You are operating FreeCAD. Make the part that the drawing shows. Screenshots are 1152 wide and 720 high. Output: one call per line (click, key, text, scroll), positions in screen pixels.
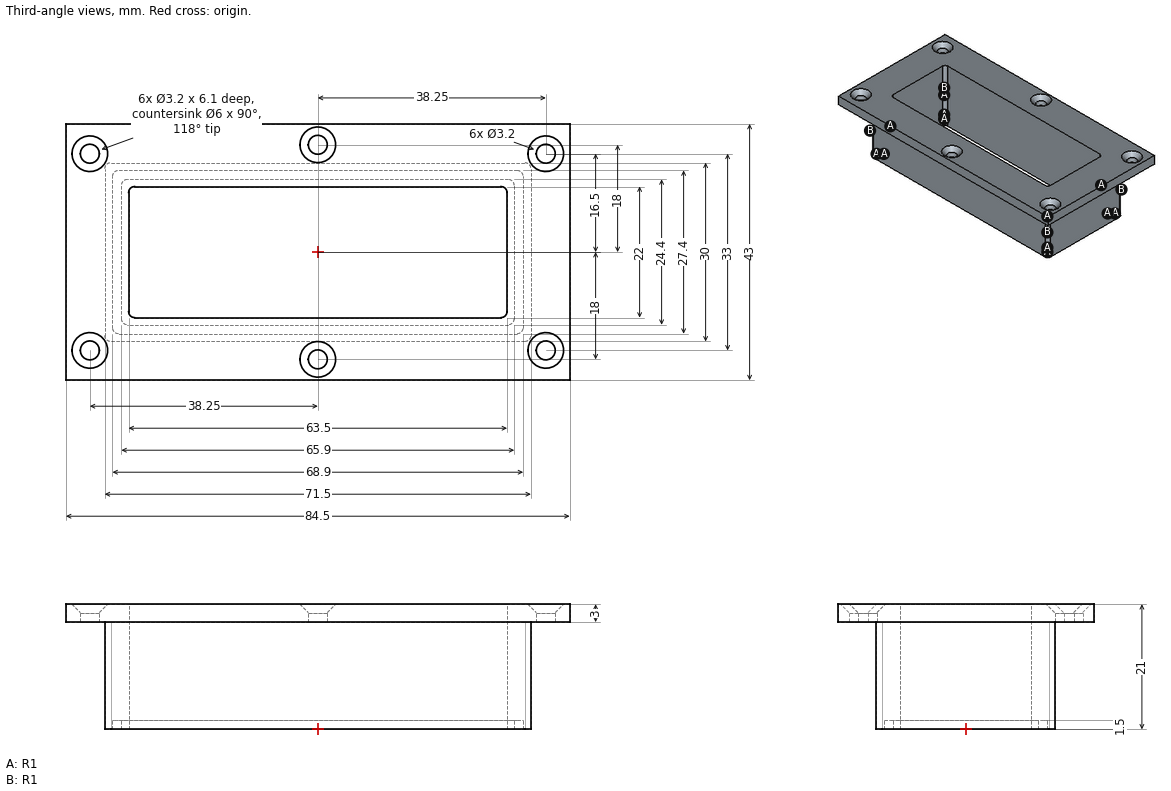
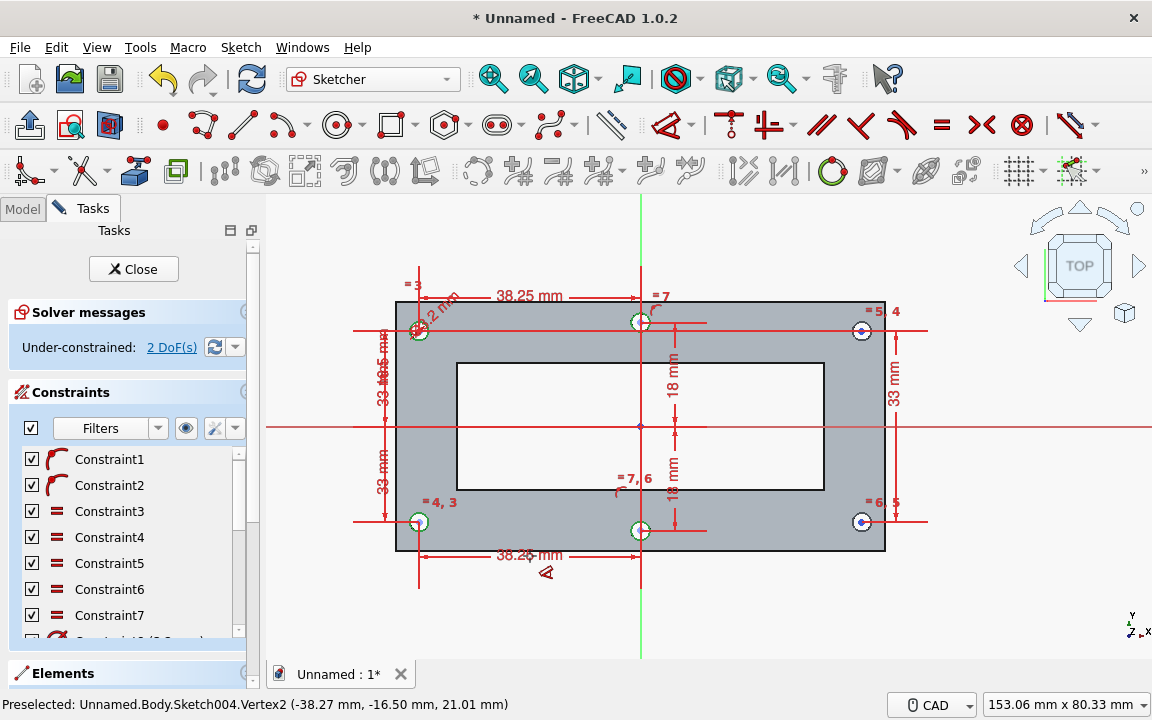
click(862, 331)
click(751, 297)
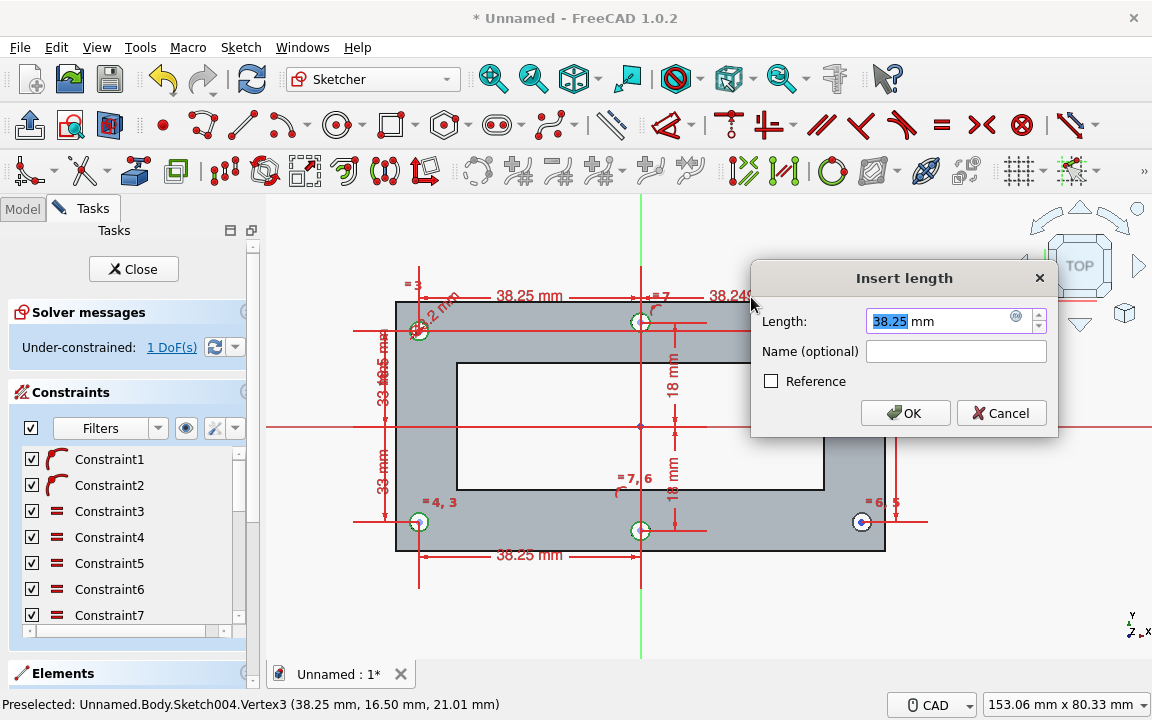
text(38.25)
key(Return)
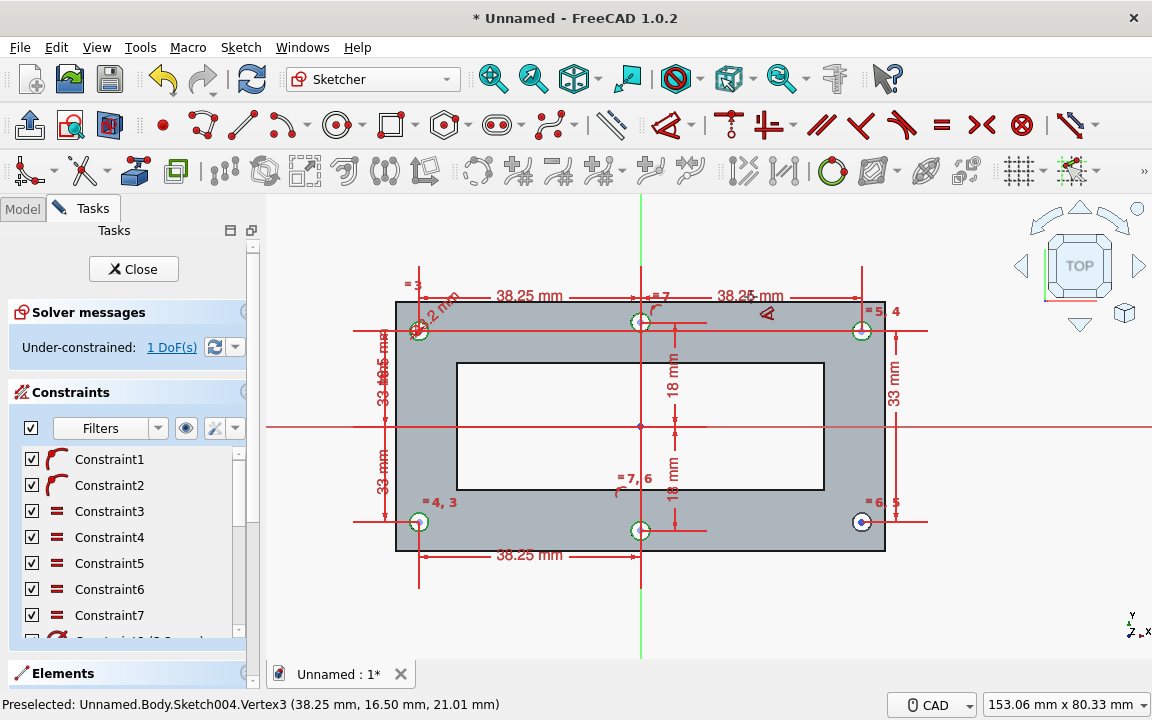
click(862, 522)
click(751, 556)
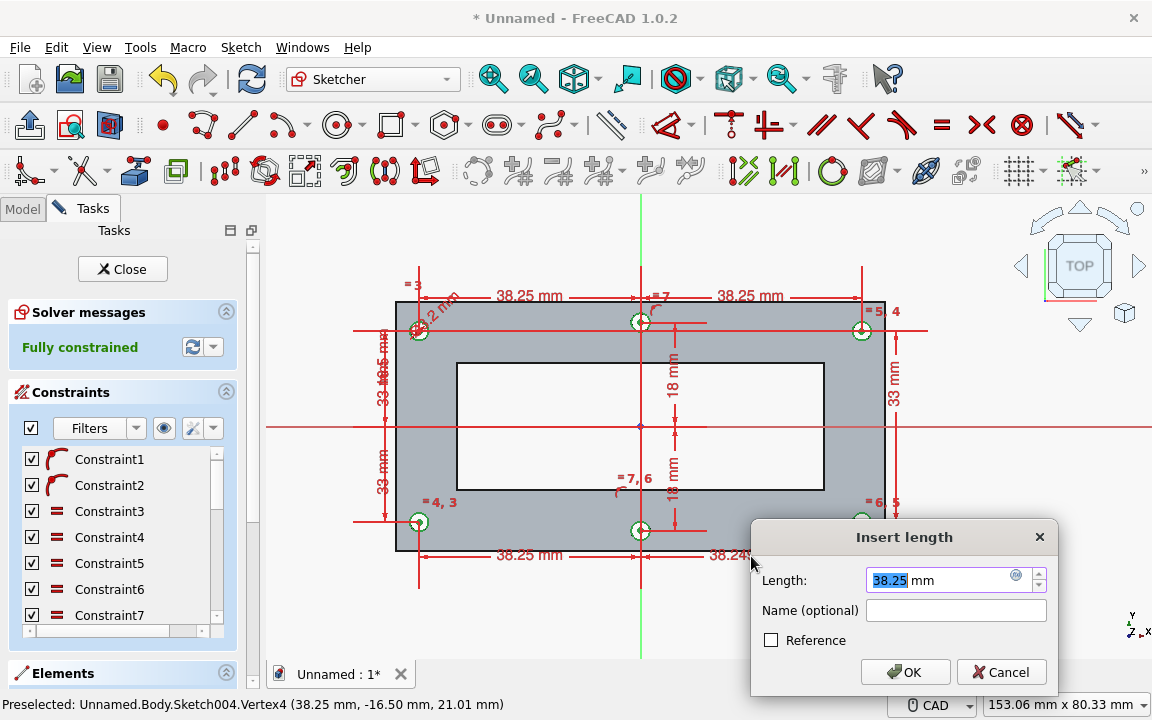
text(38.25)
key(Return)
key(Escape)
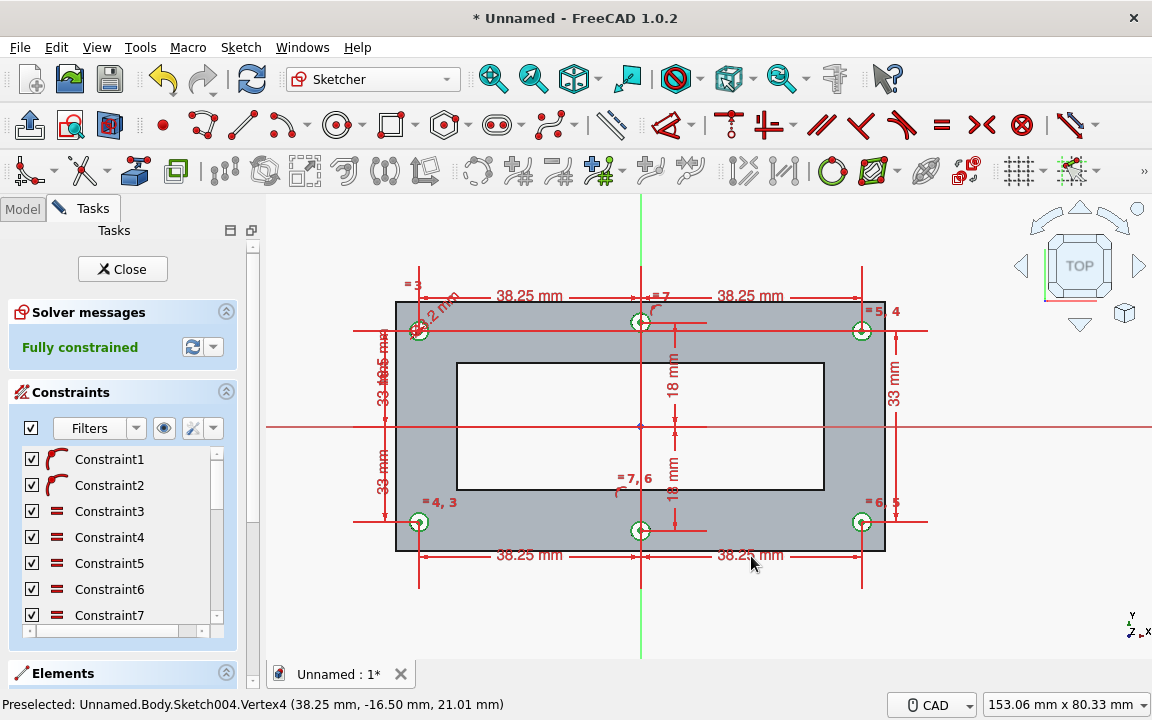
click(123, 269)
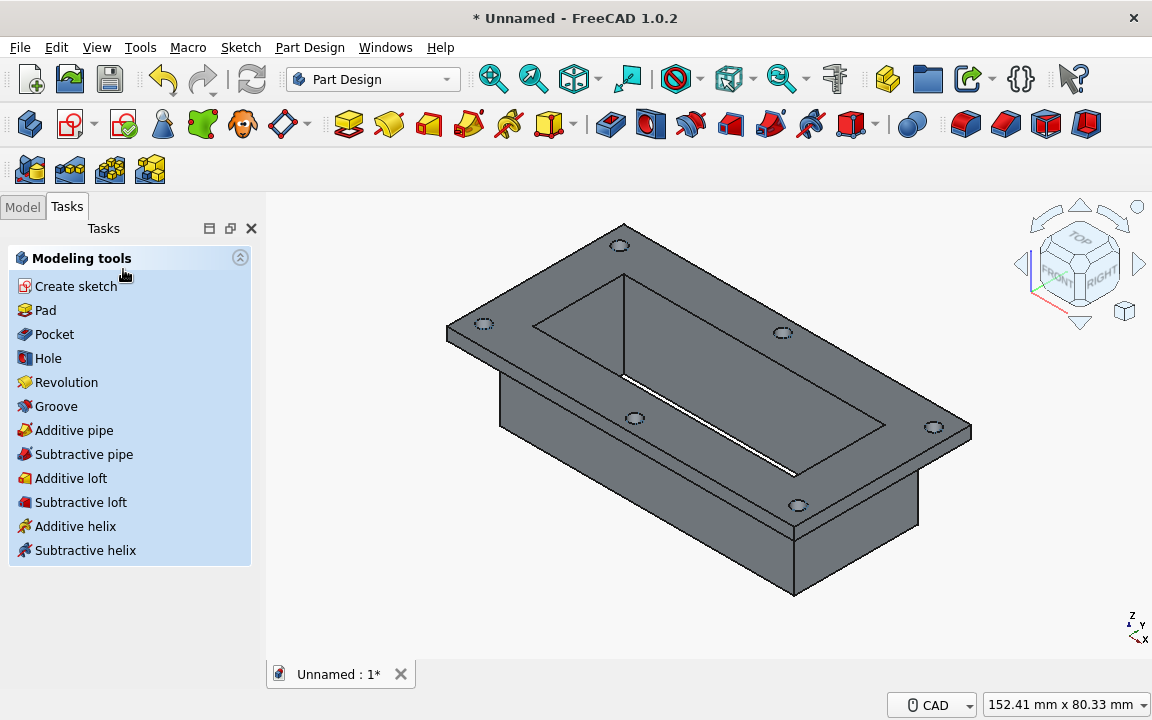
click(652, 124)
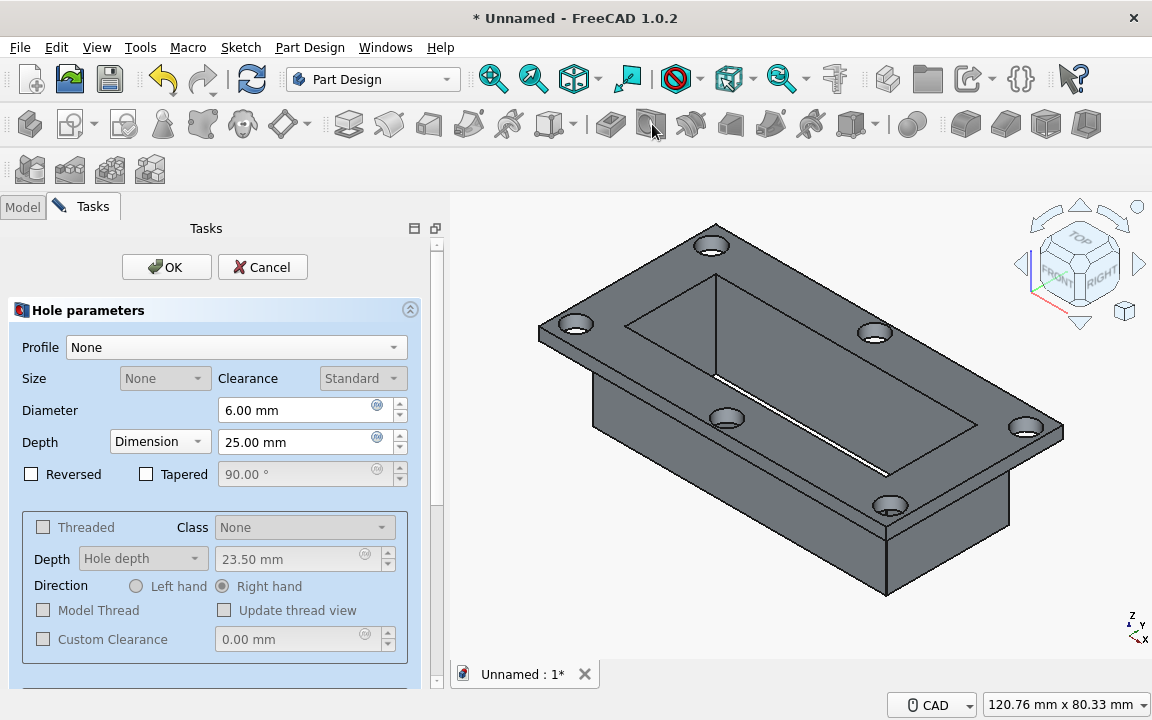
triple_click(305, 410)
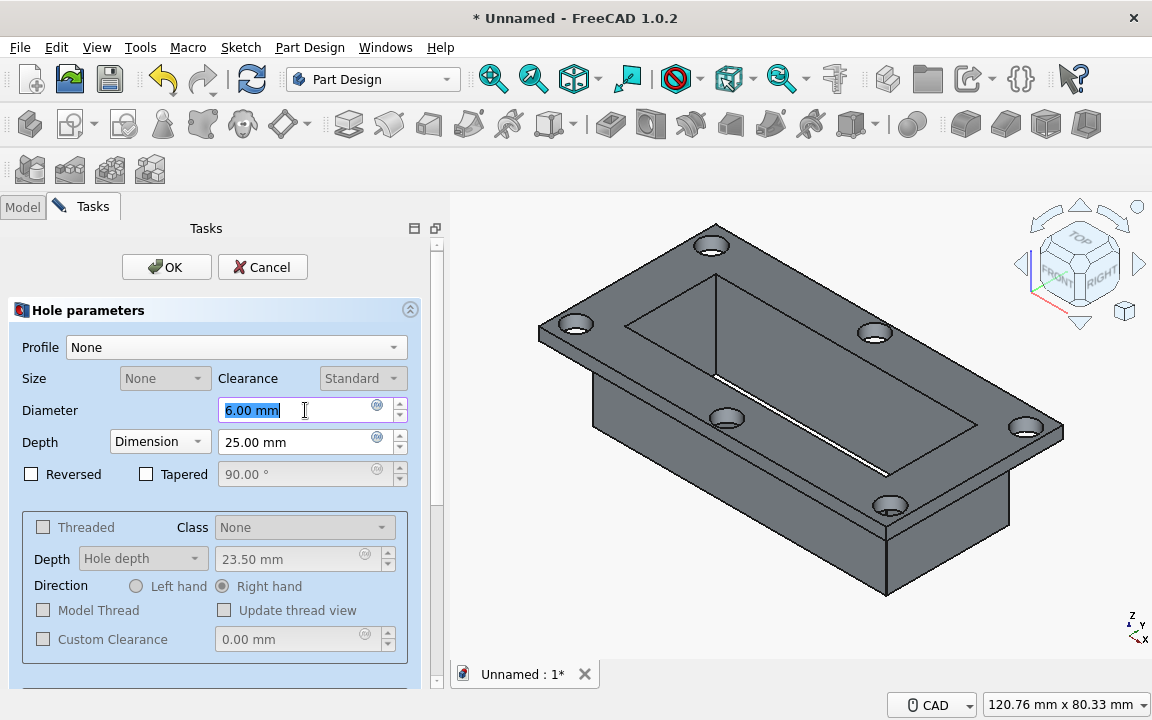
text(3.2)
key(Tab)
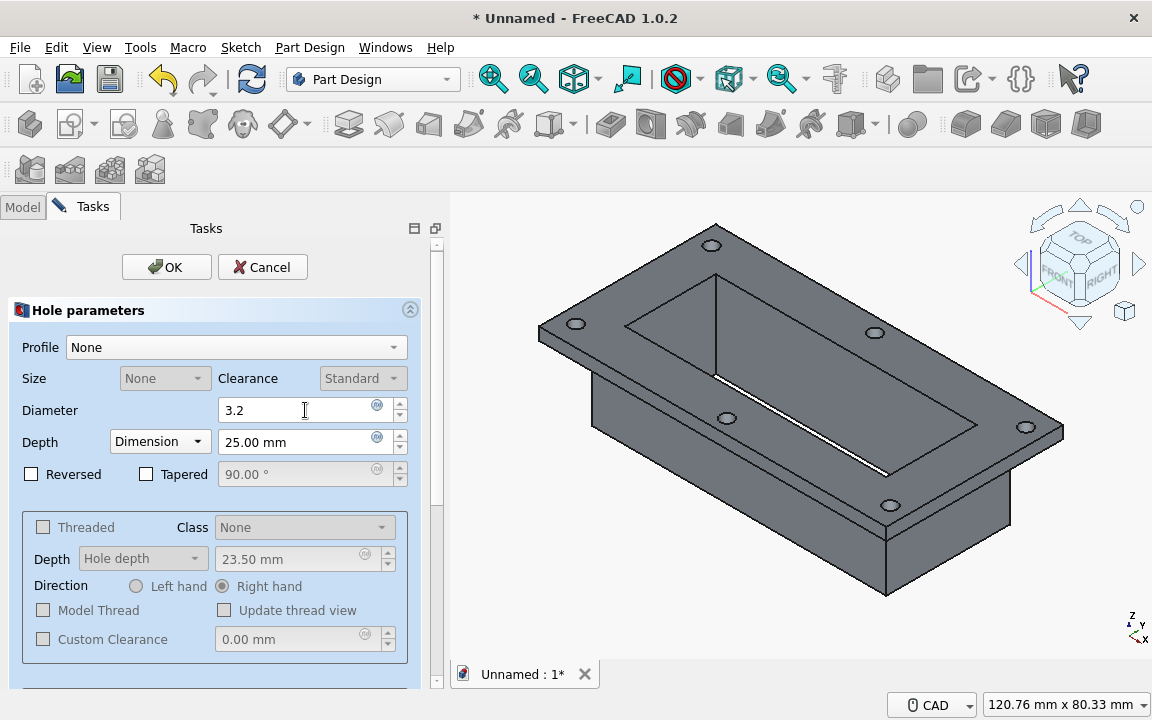
triple_click(305, 442)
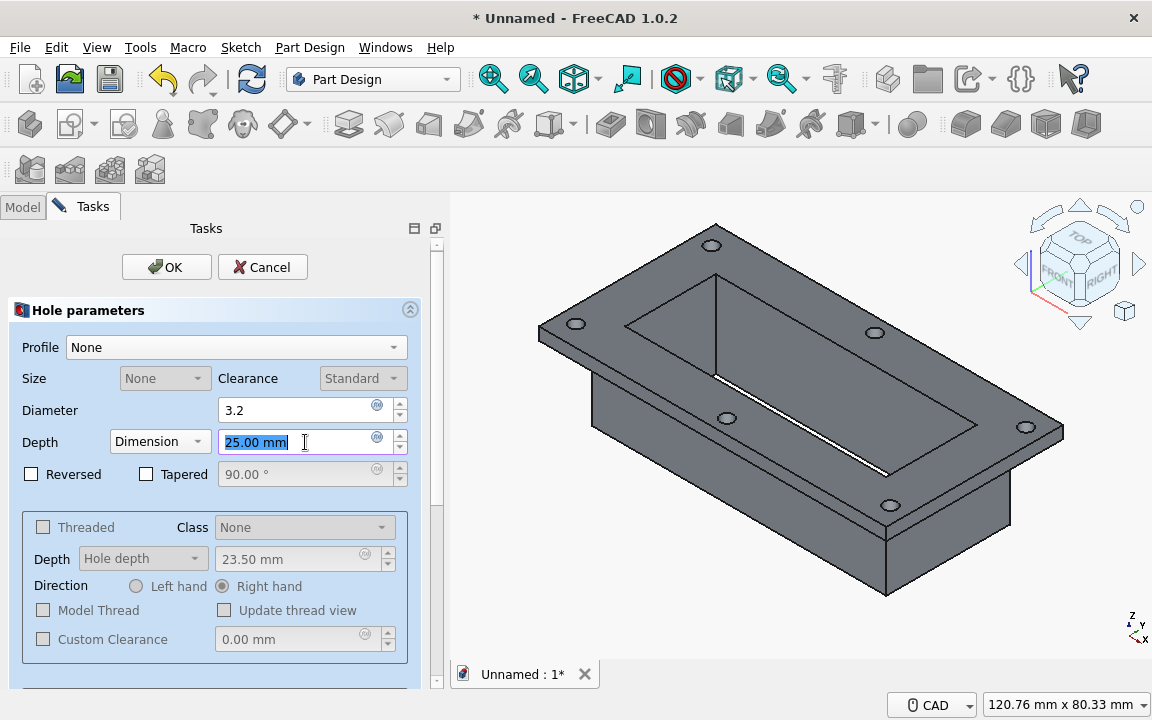
text(6.1)
key(Tab)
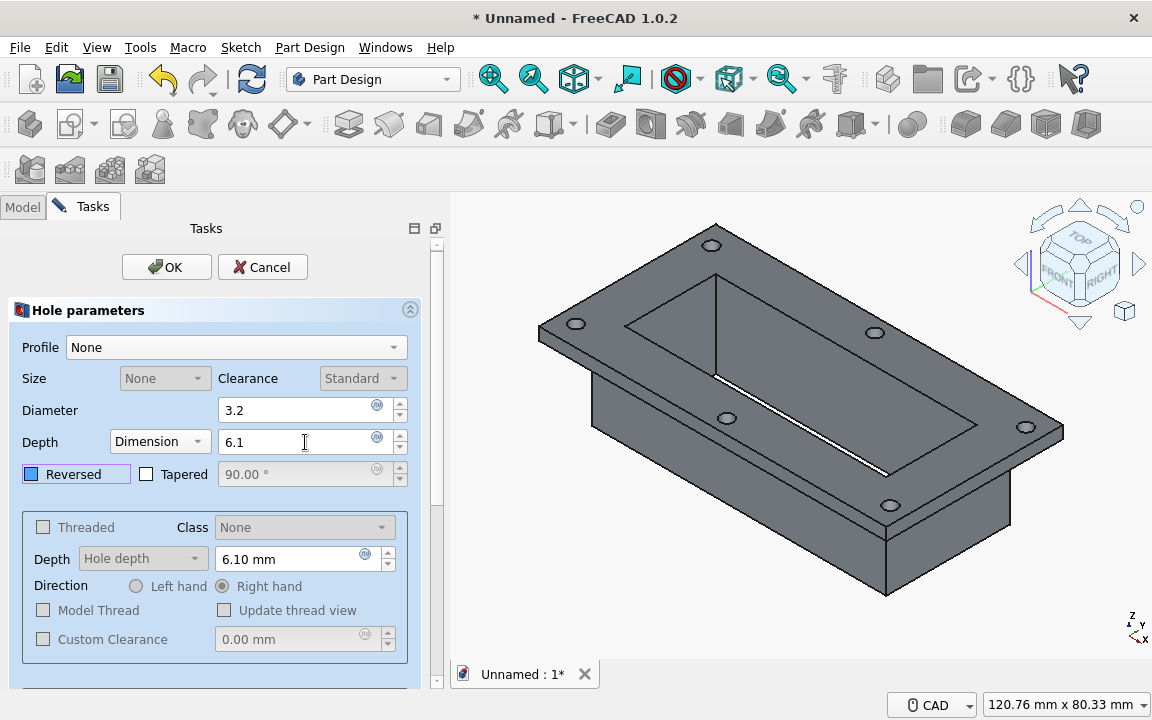
scroll(437, 463, down, 2)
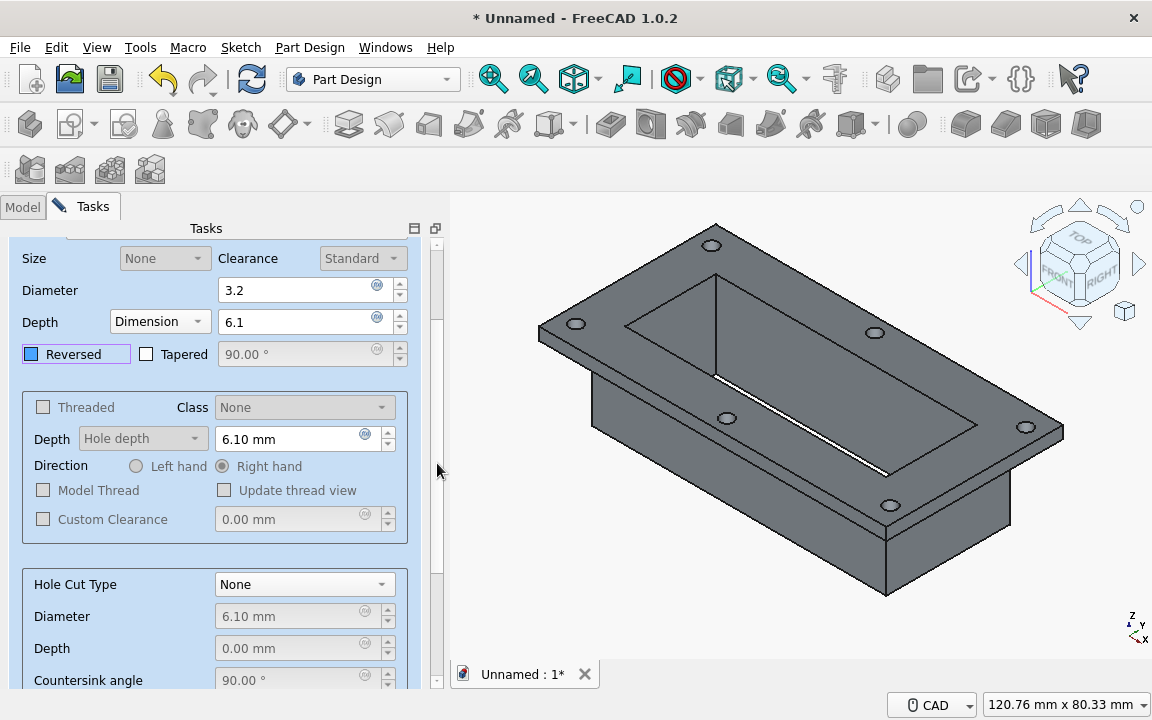
click(306, 584)